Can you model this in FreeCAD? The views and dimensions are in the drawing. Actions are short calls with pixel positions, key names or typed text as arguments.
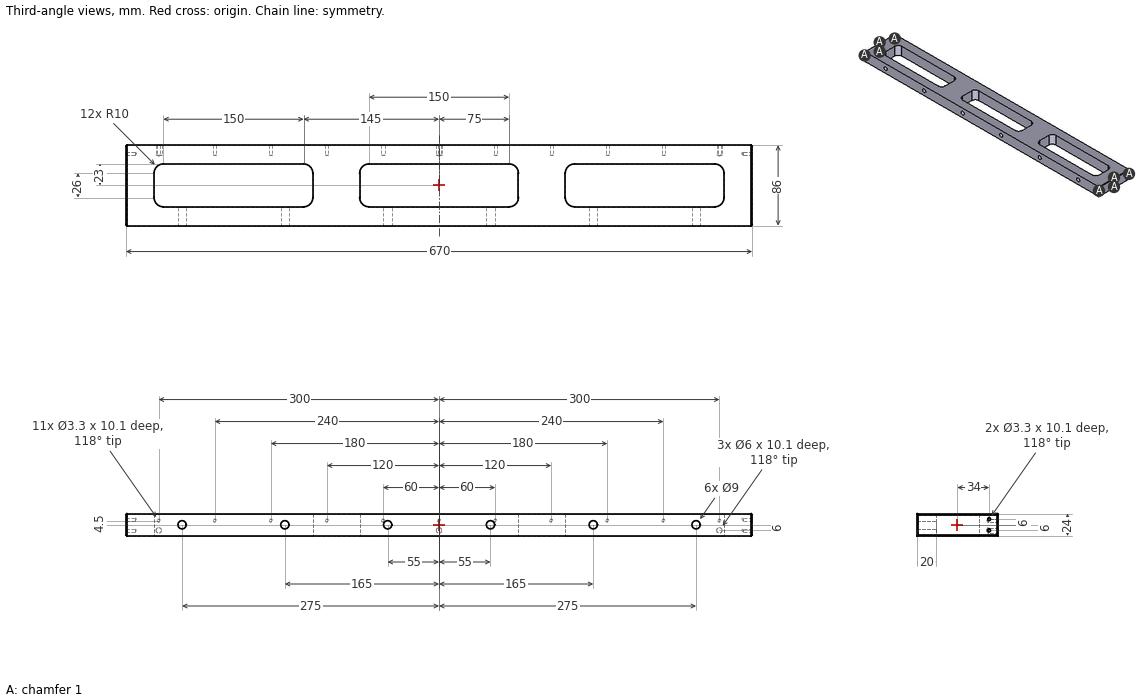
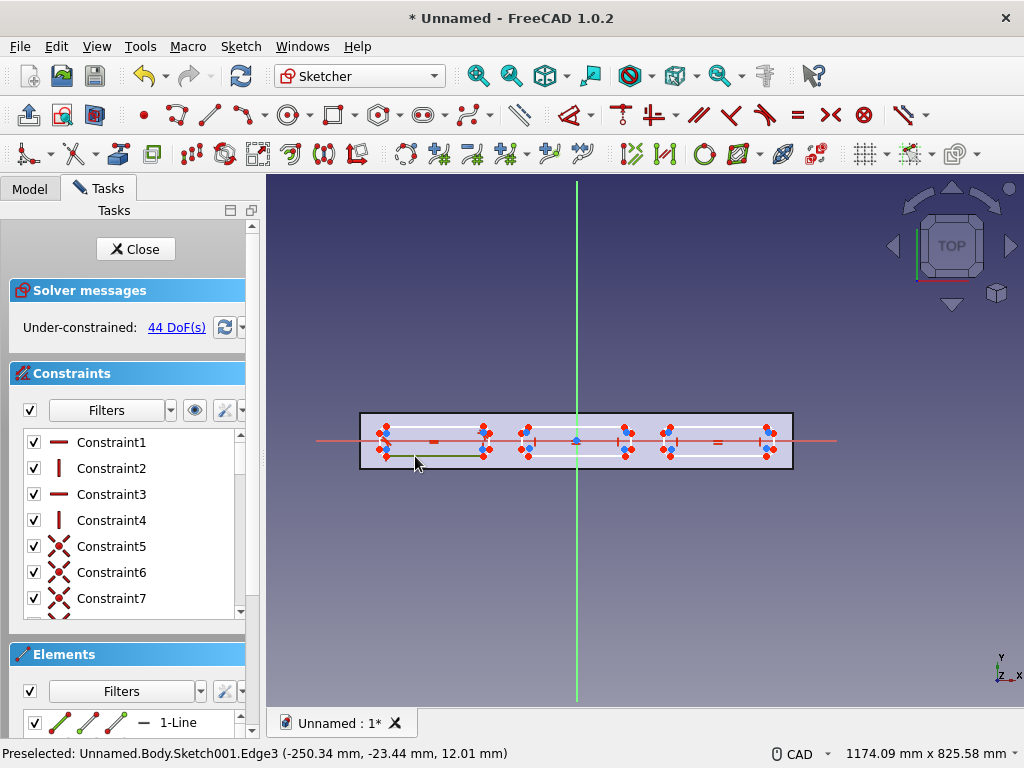
scroll(382, 454, up, 6)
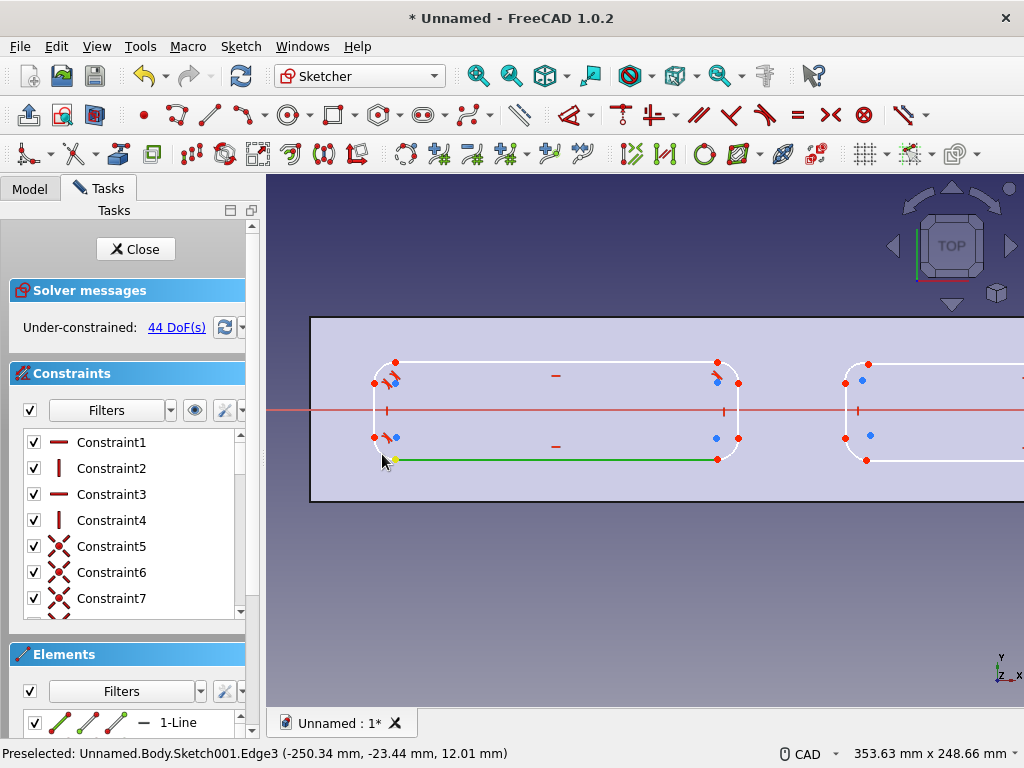
click(380, 453)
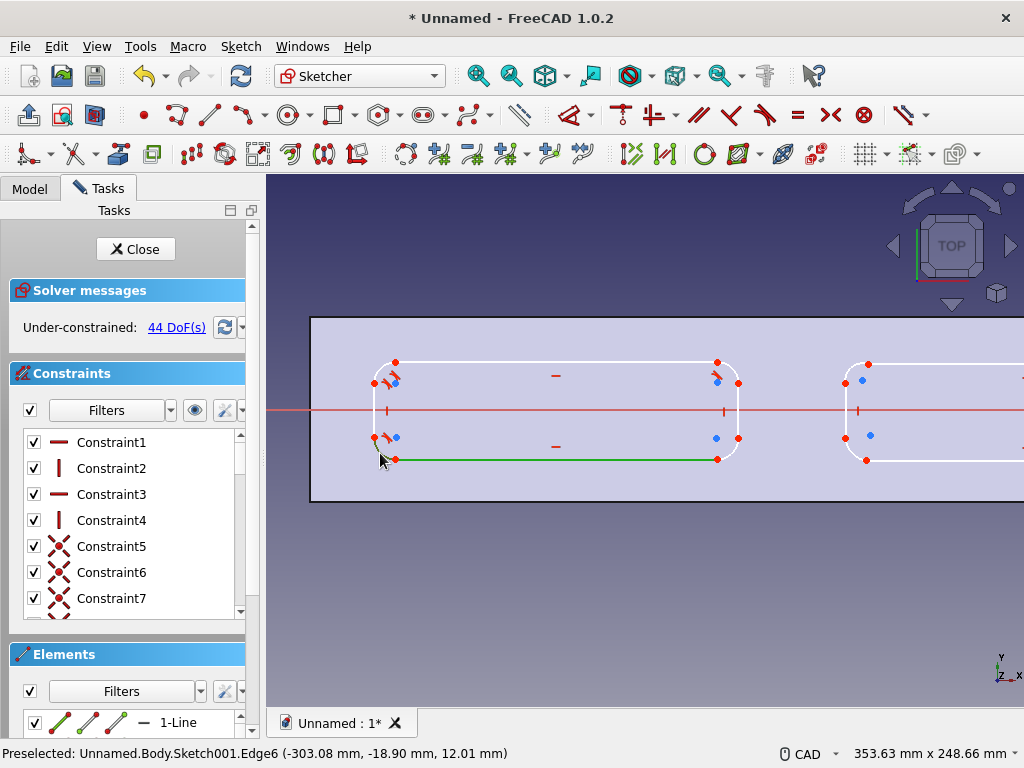
key(t)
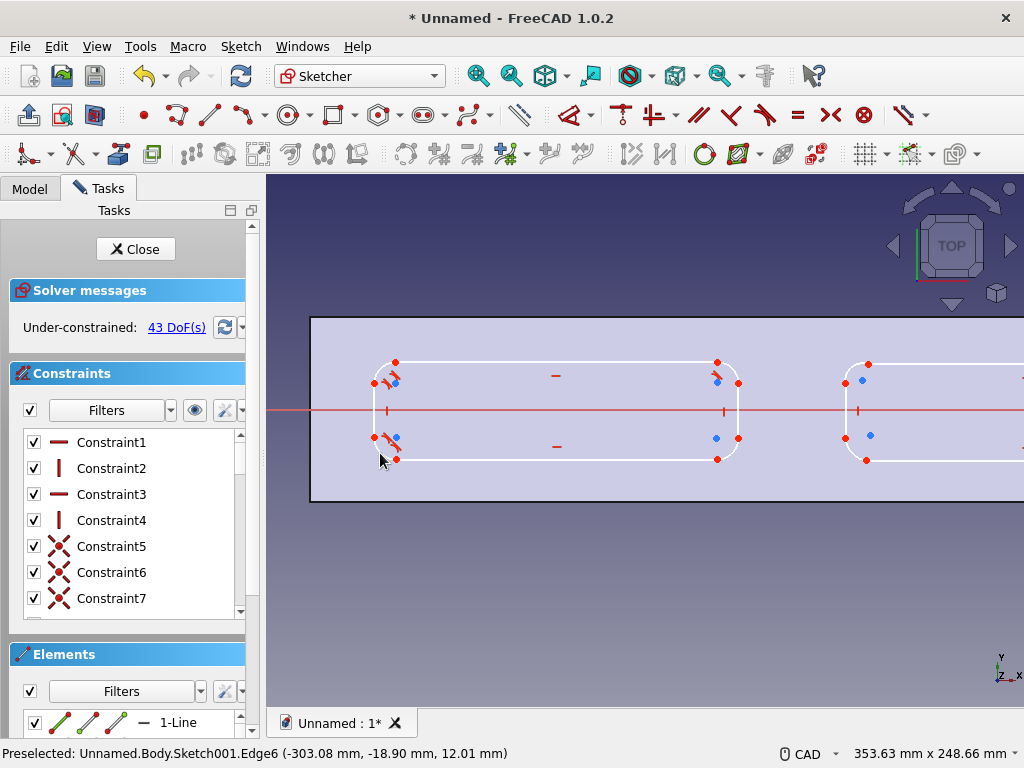
click(493, 460)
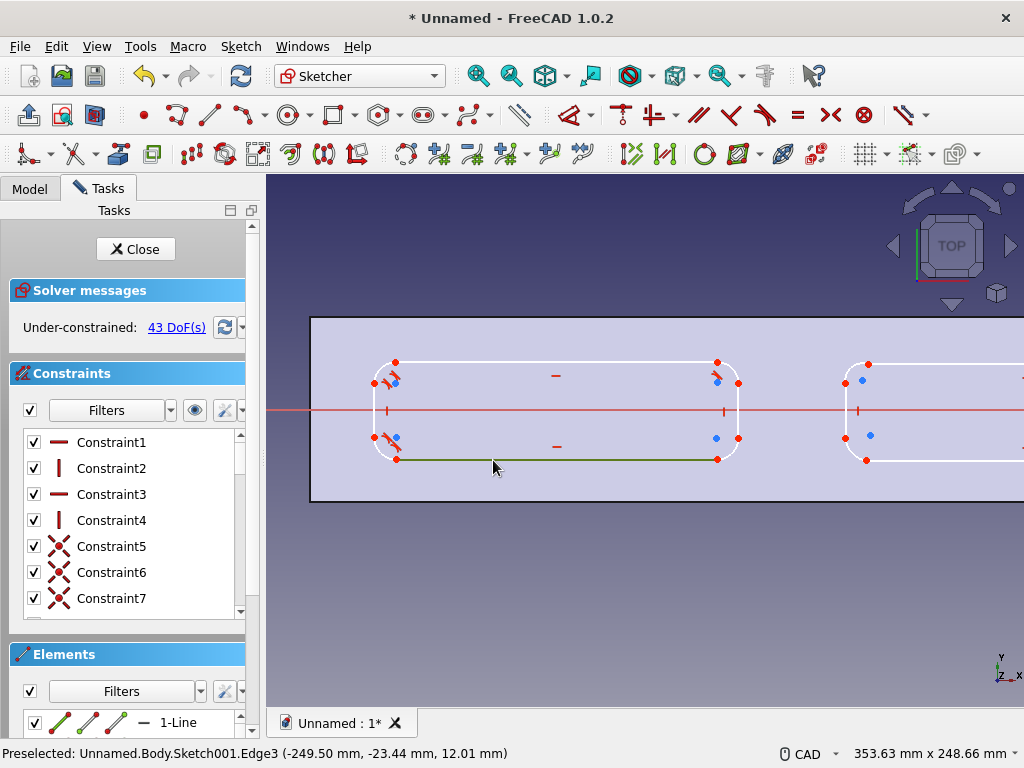
scroll(727, 457, up, 2)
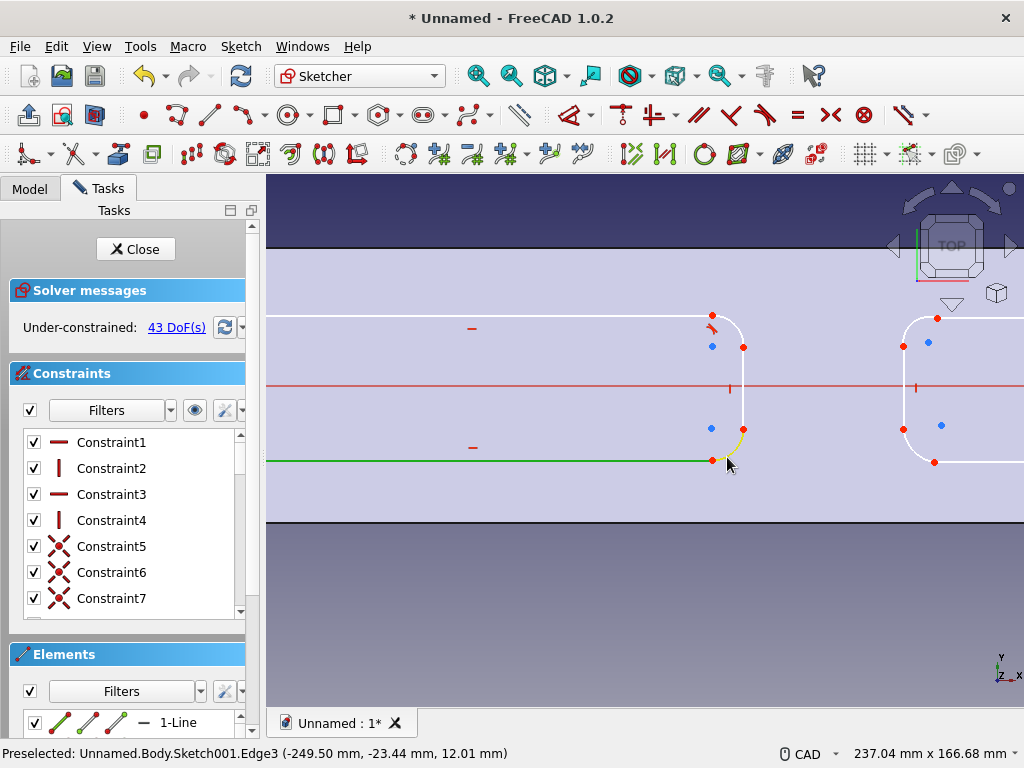
click(726, 457)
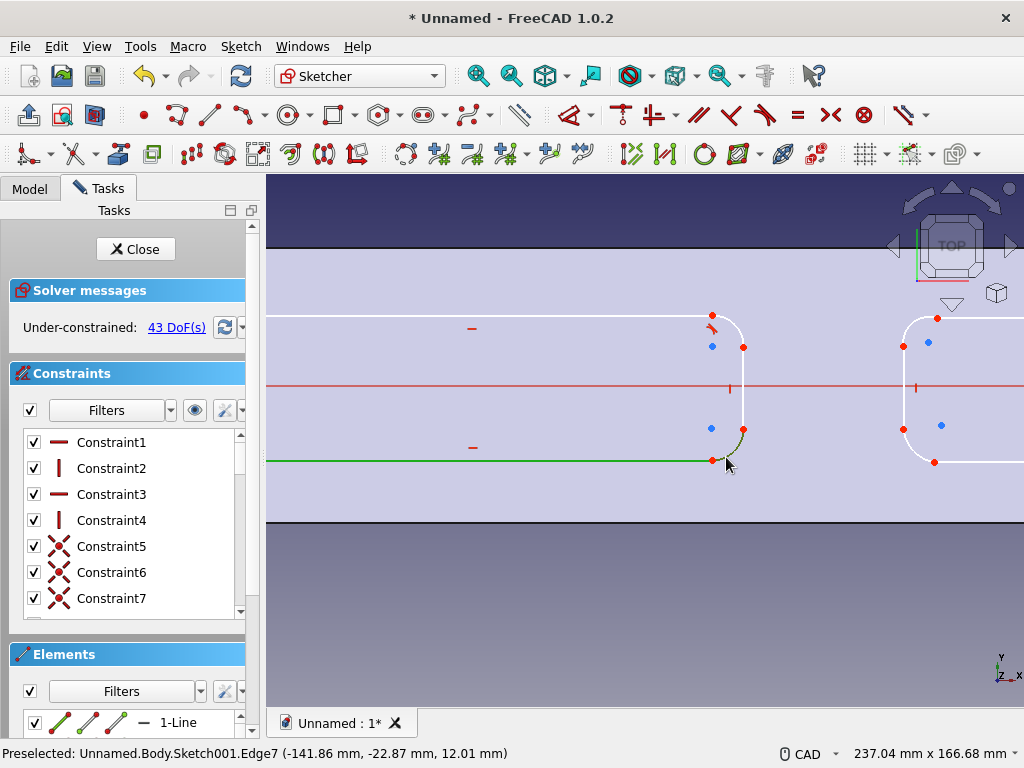
click(765, 116)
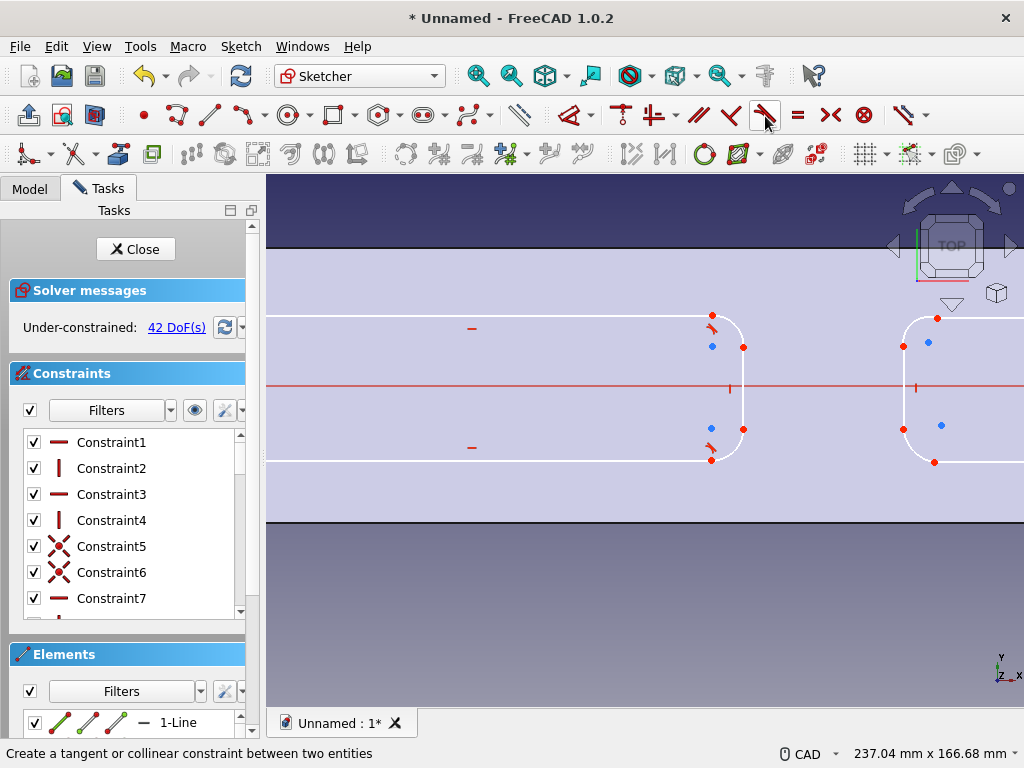
click(743, 405)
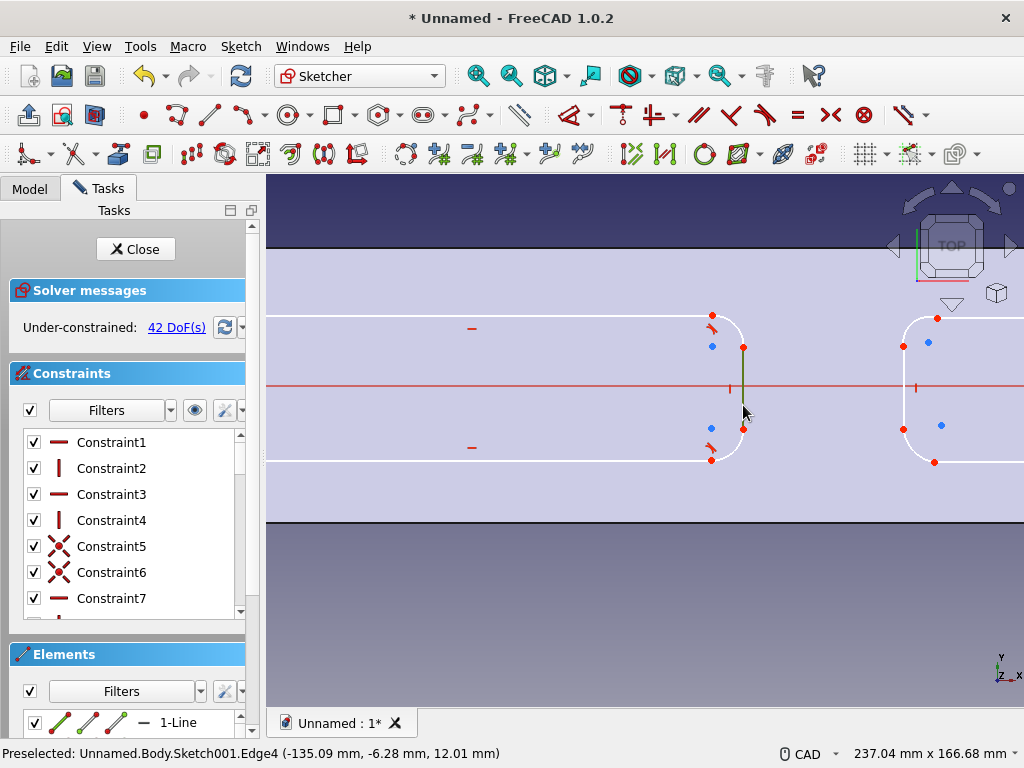
click(725, 458)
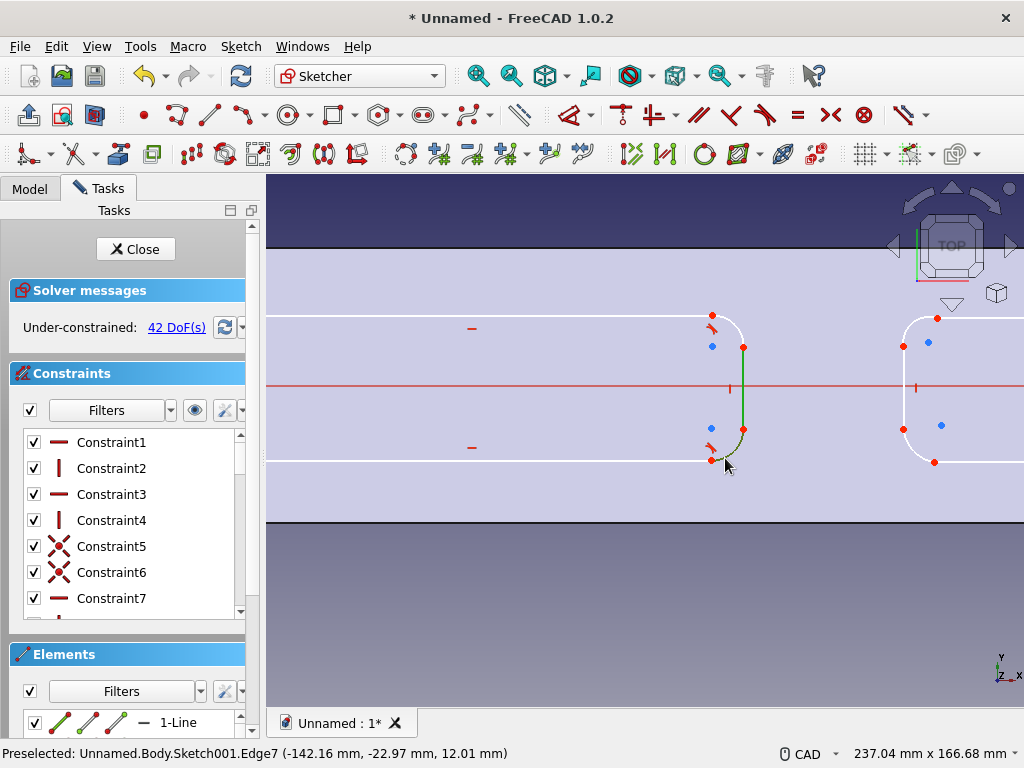
key(t)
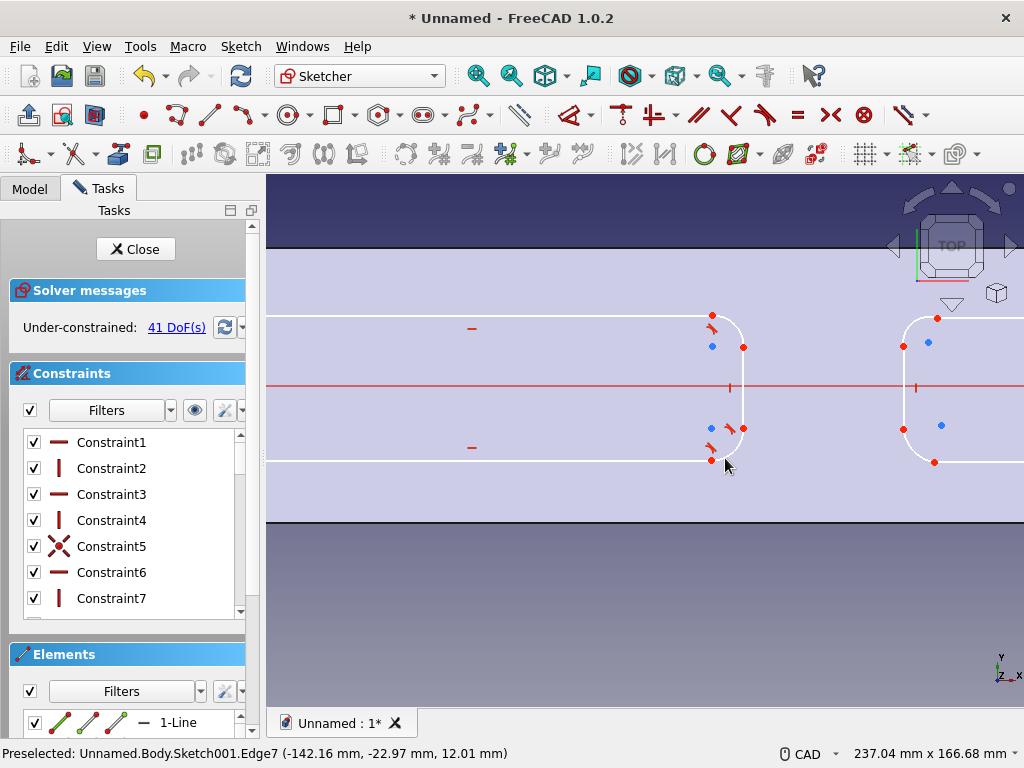
click(743, 404)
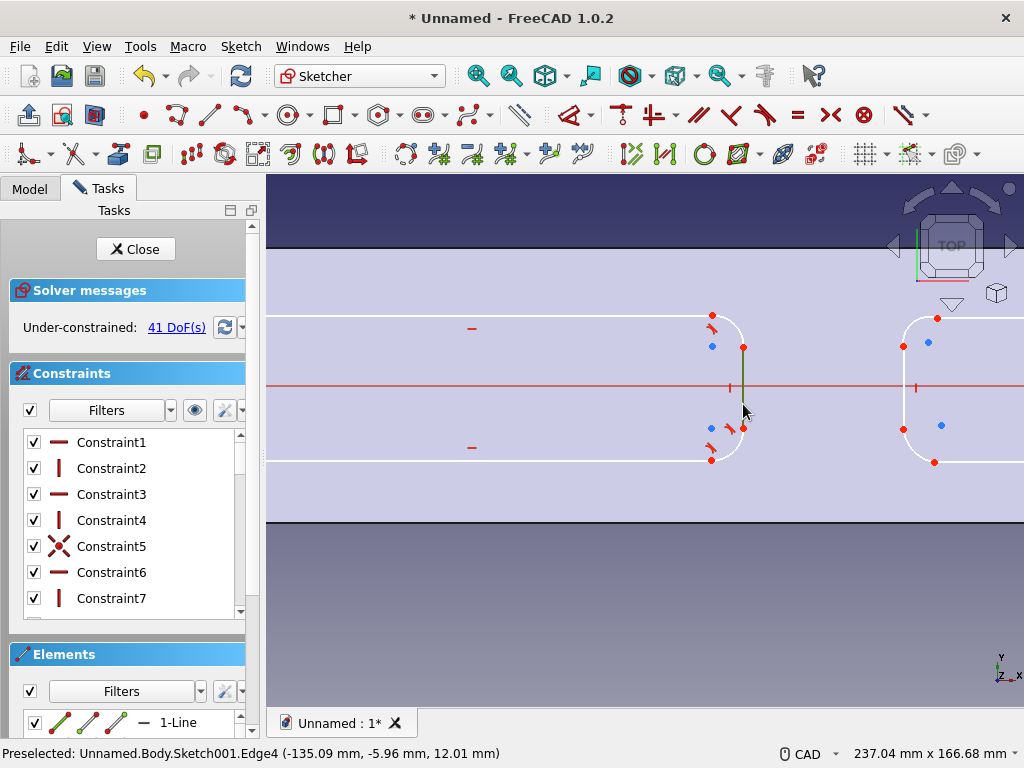
click(741, 333)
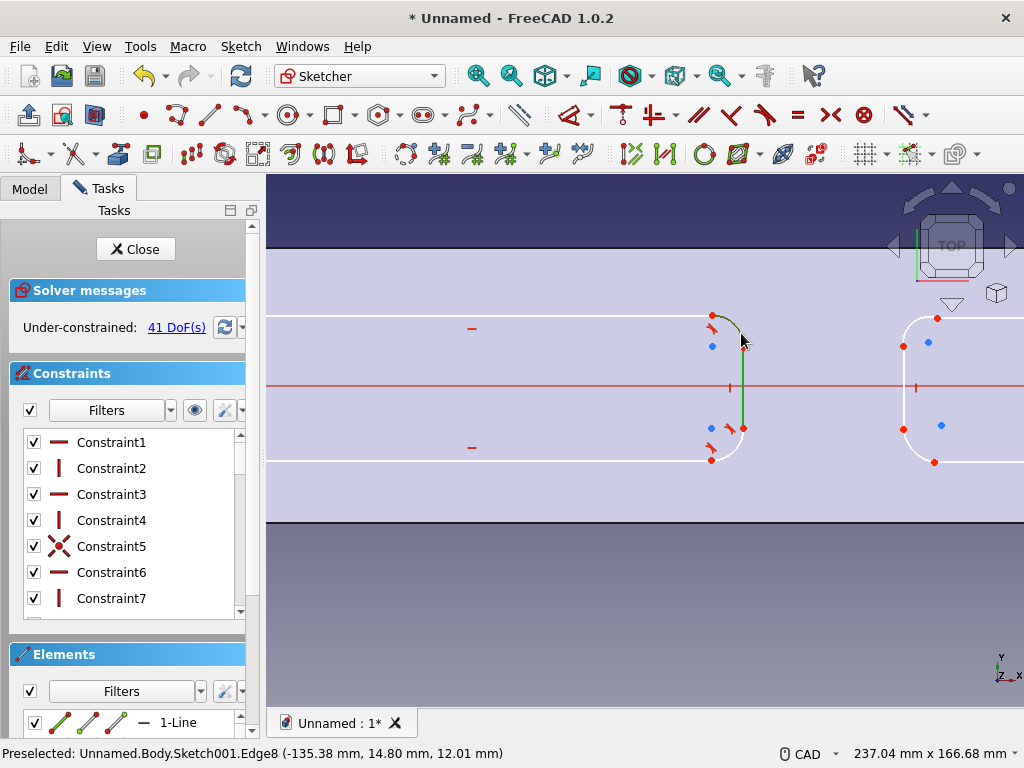
click(765, 116)